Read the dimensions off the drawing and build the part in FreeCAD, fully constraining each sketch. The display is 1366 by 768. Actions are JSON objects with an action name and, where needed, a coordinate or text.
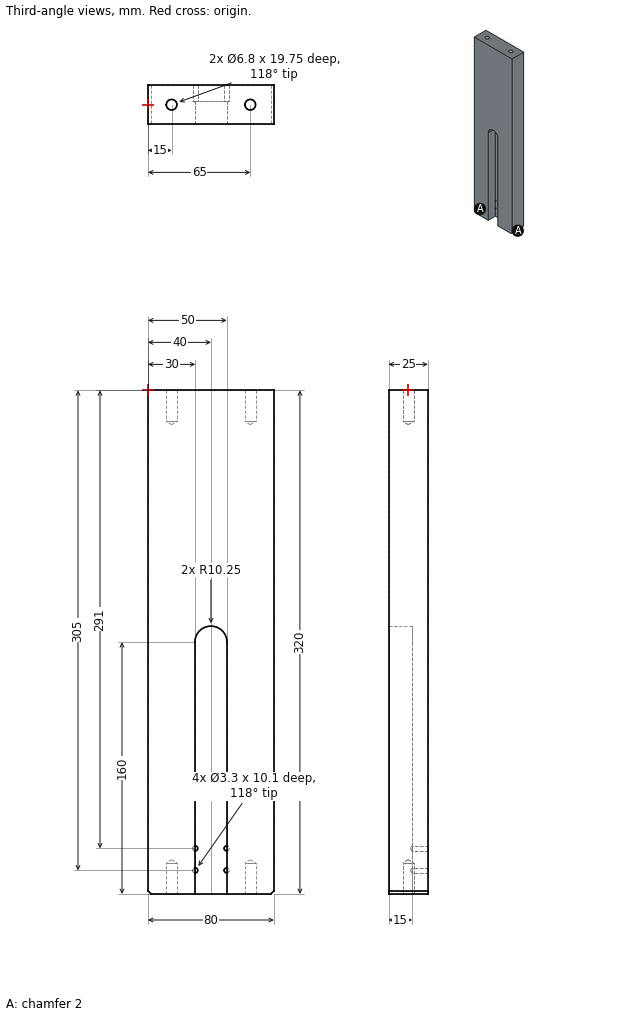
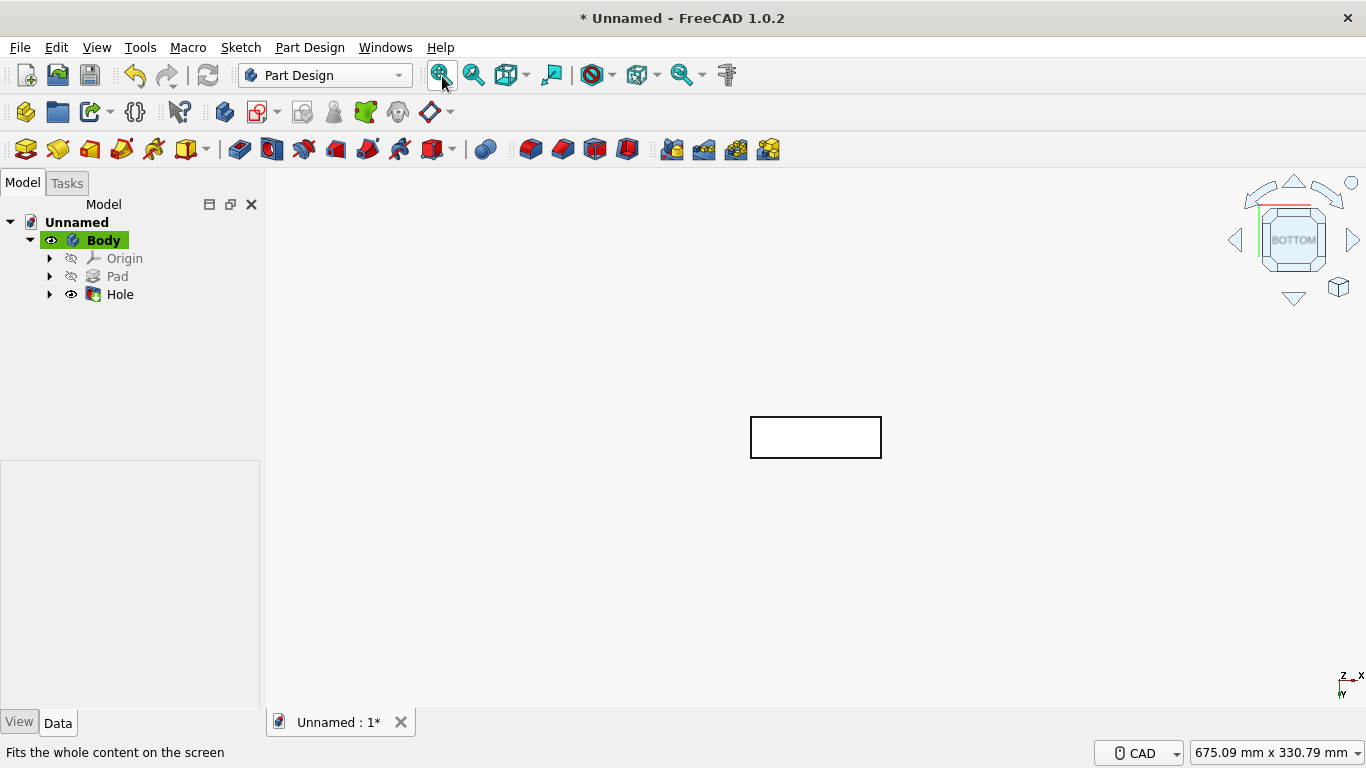
{"action": "key", "text": "v f"}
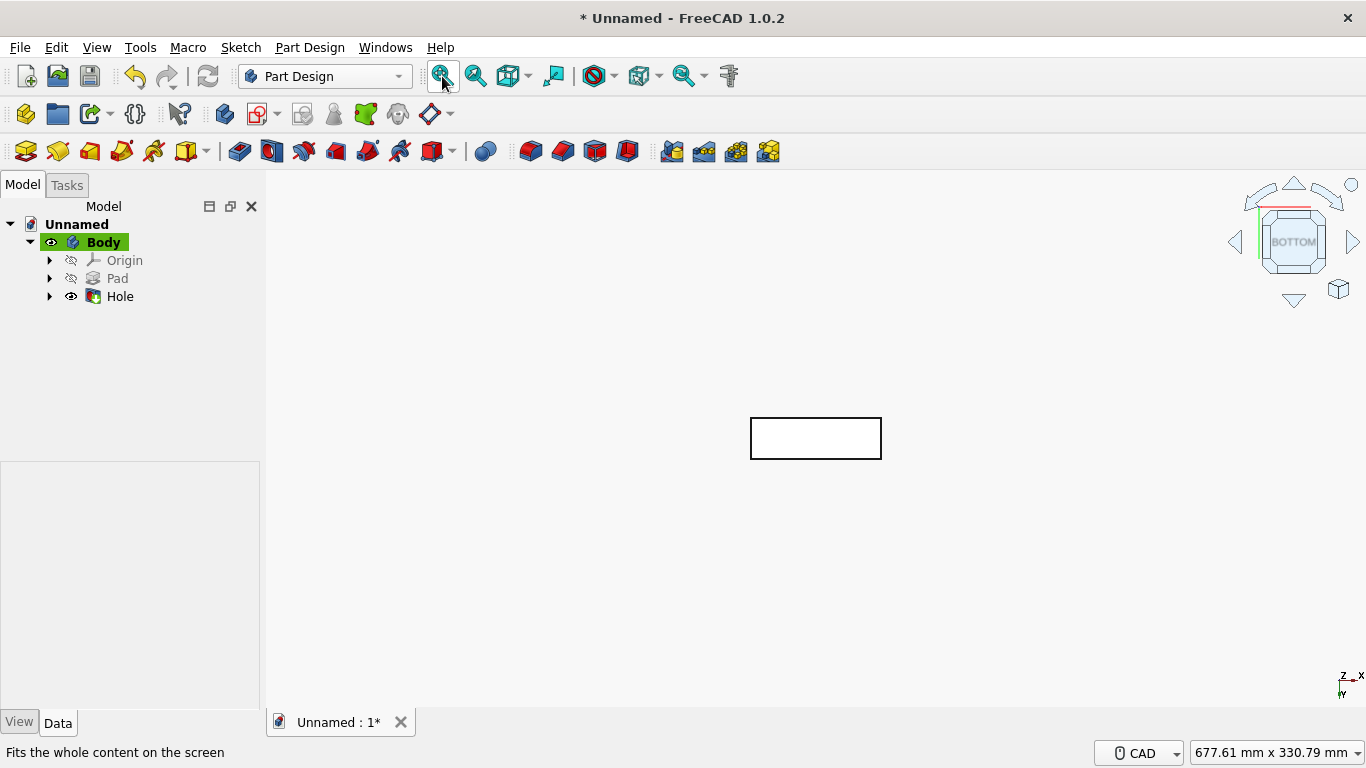
{"action": "left_click", "coordinate": [751, 437]}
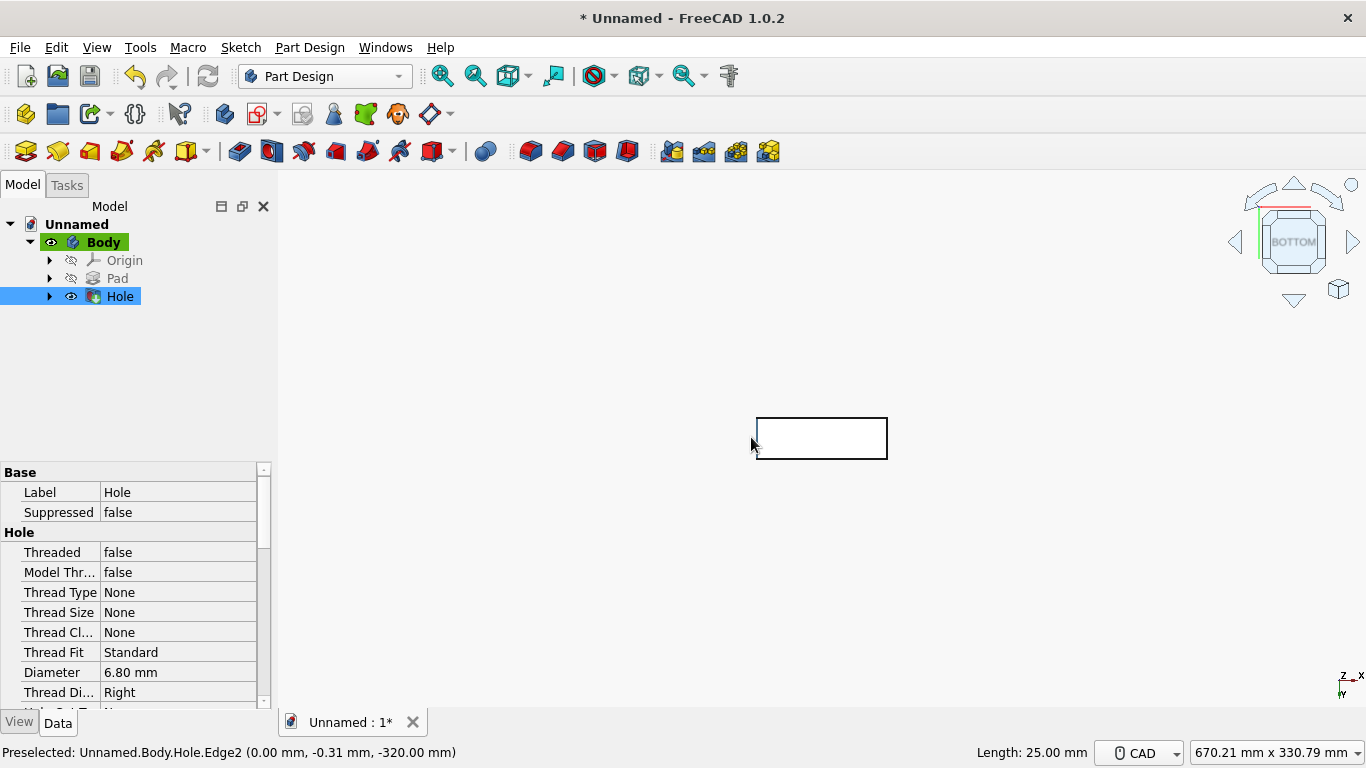
{"action": "left_click", "coordinate": [887, 437], "text": "ctrl"}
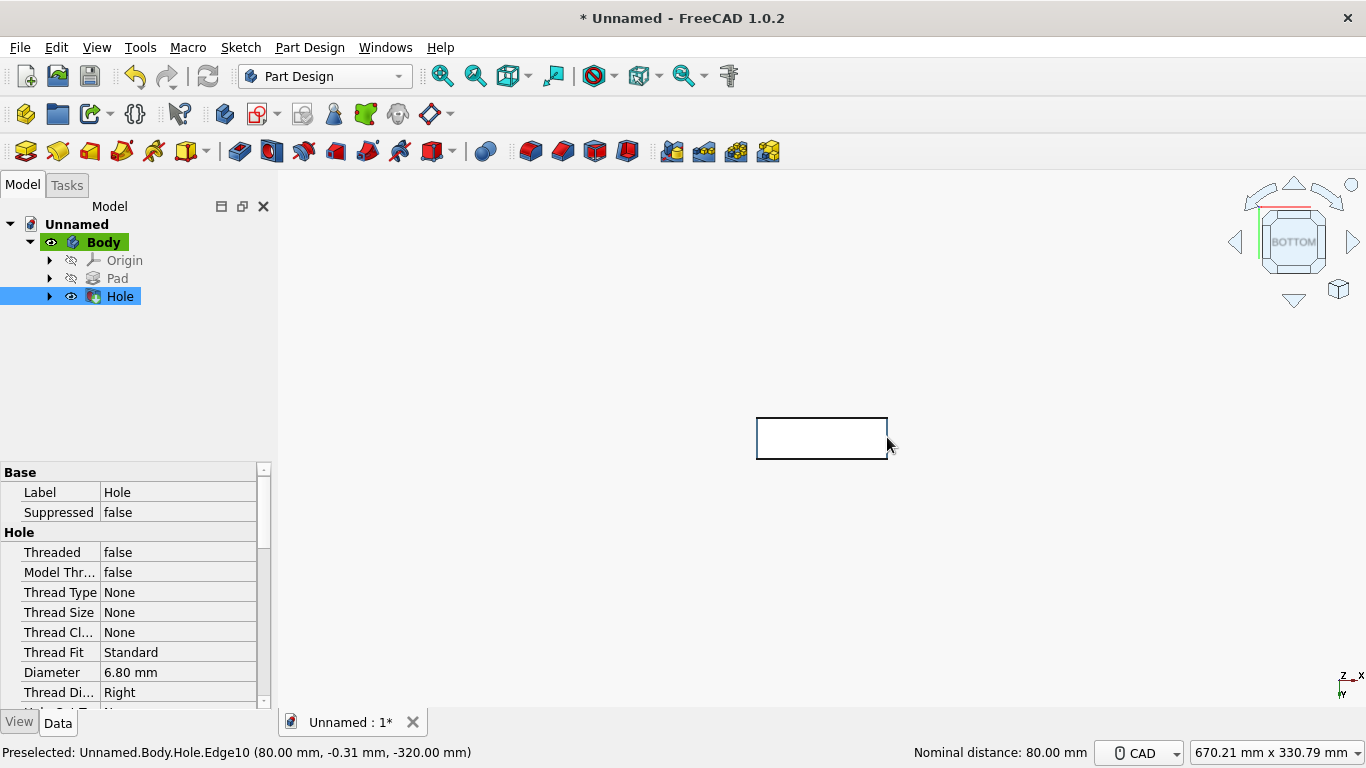
{"action": "left_click", "coordinate": [564, 152]}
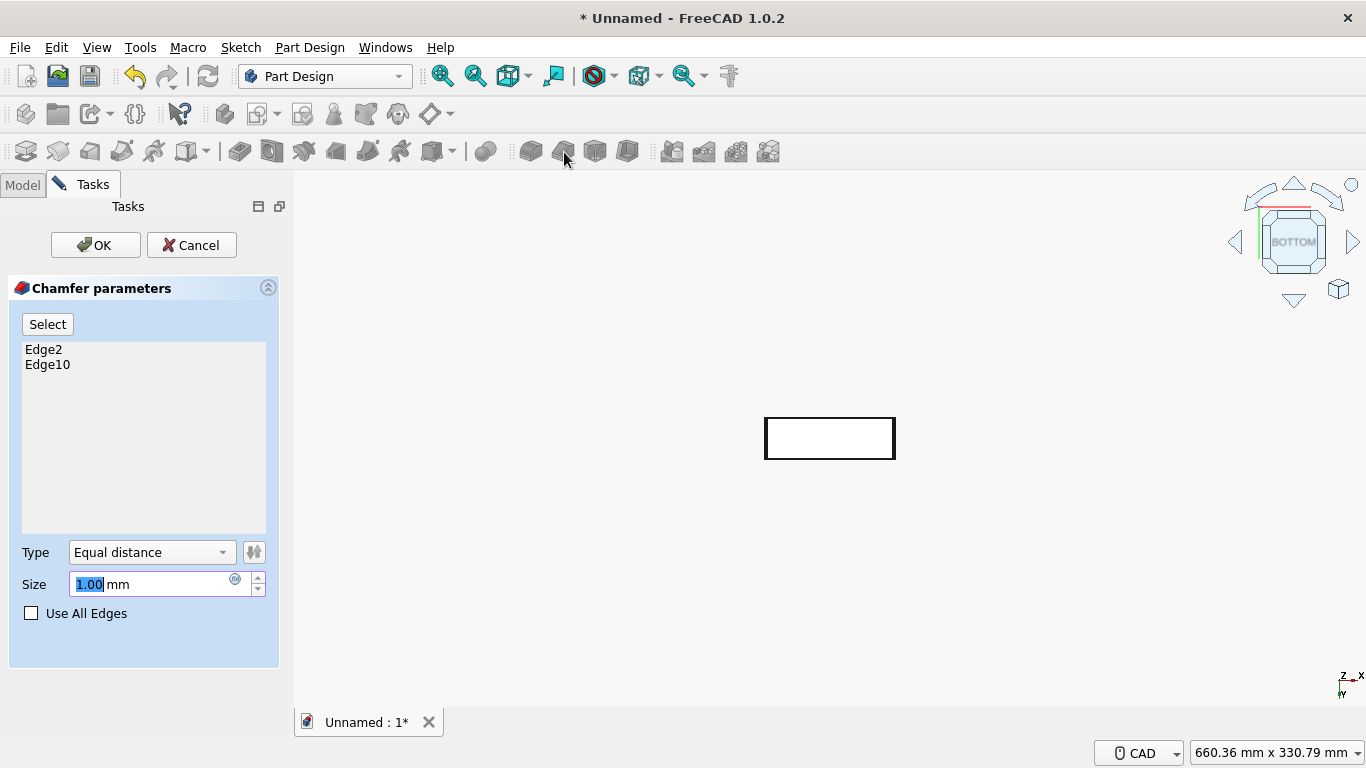
{"action": "type", "text": "2"}
{"action": "key", "text": "Tab"}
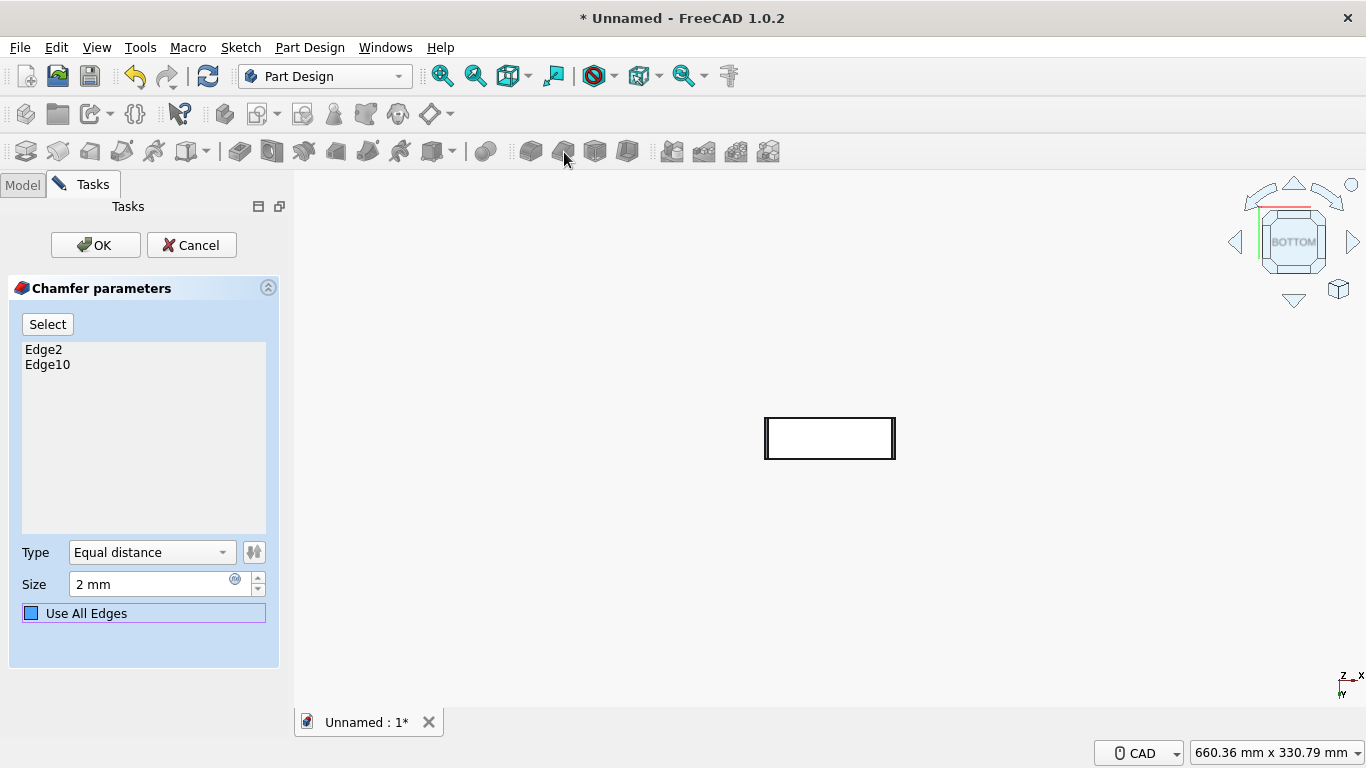
{"action": "left_click", "coordinate": [96, 245]}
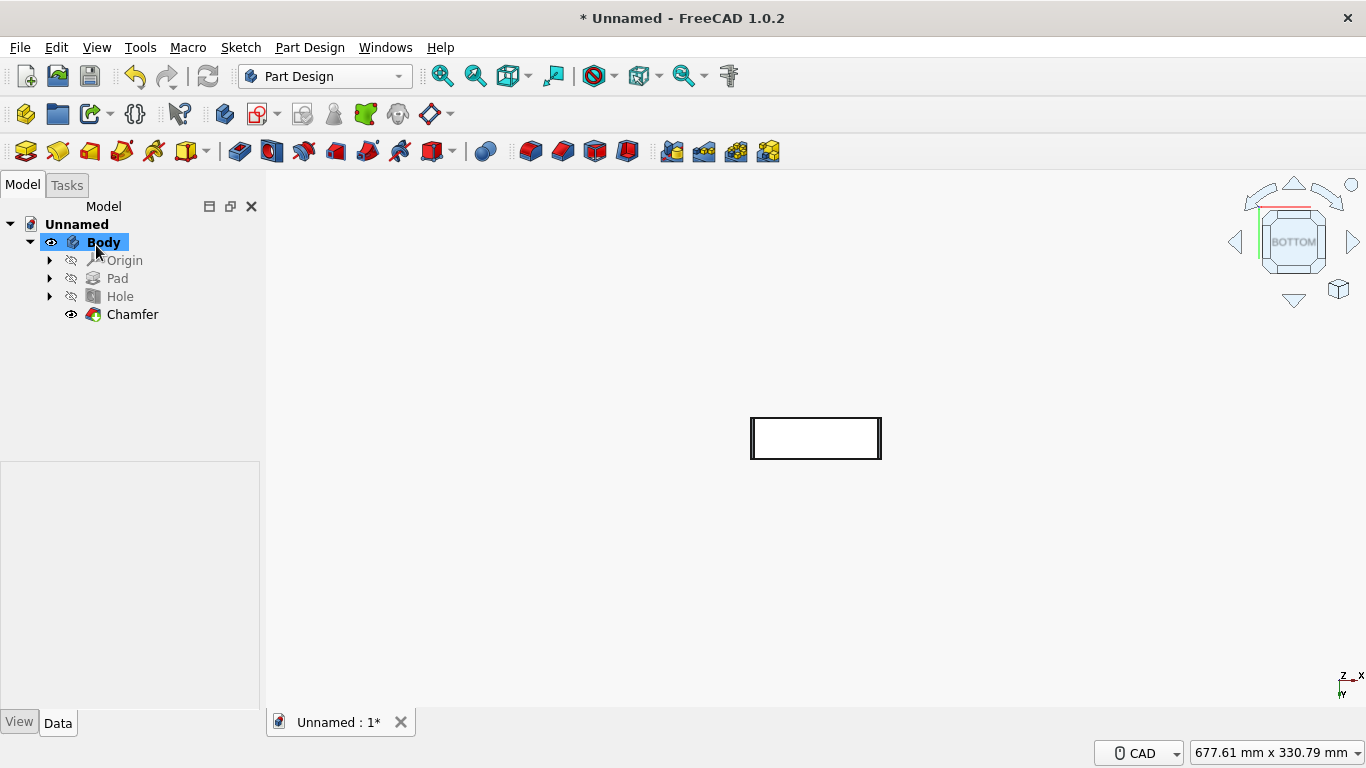
{"action": "key", "text": "v f"}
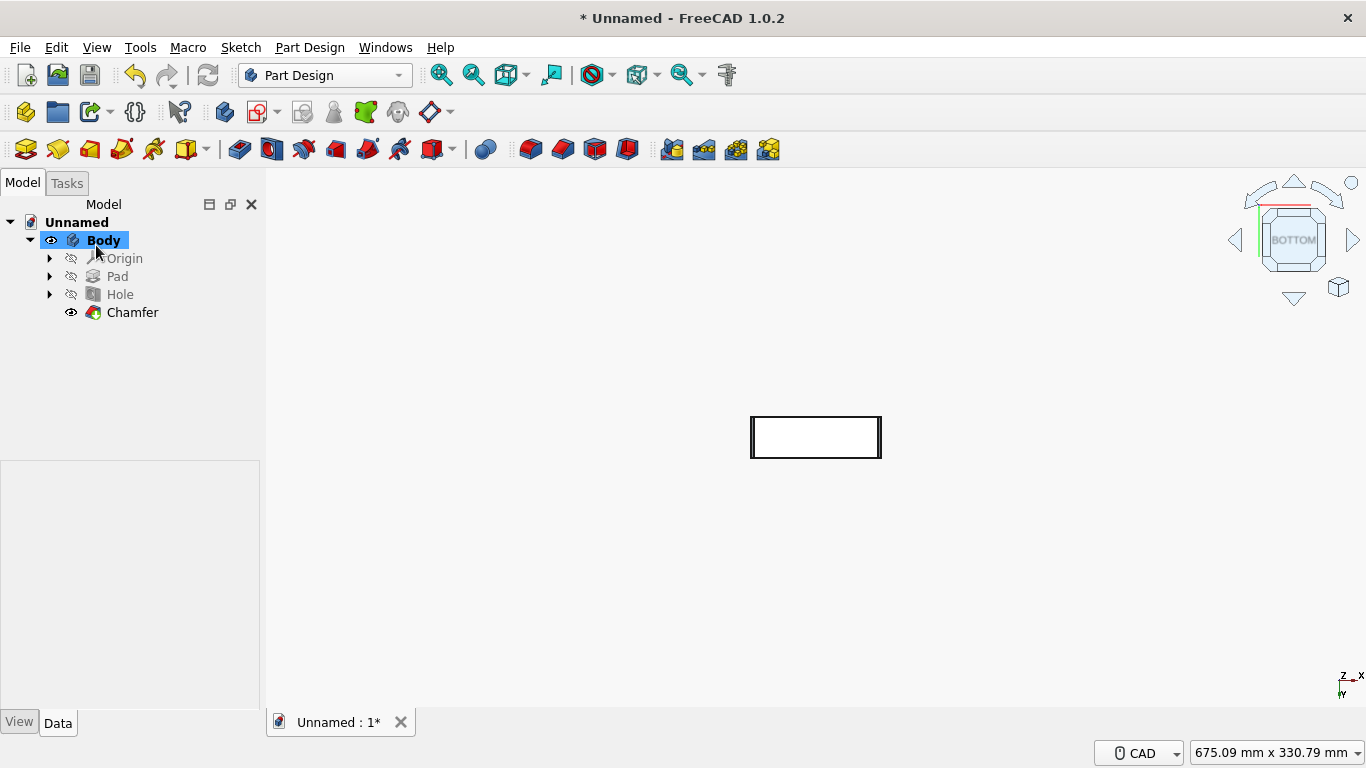
{"action": "key", "text": "4"}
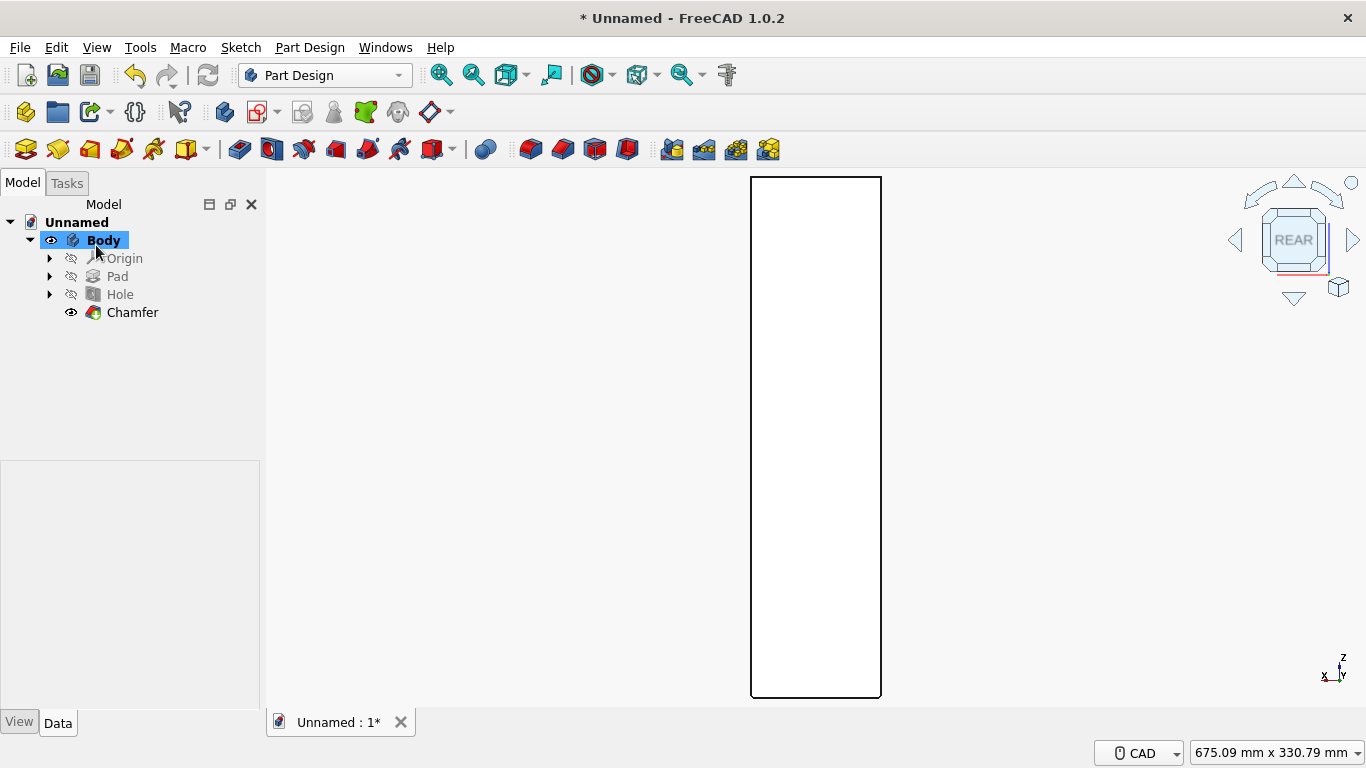
{"action": "left_click", "coordinate": [816, 288]}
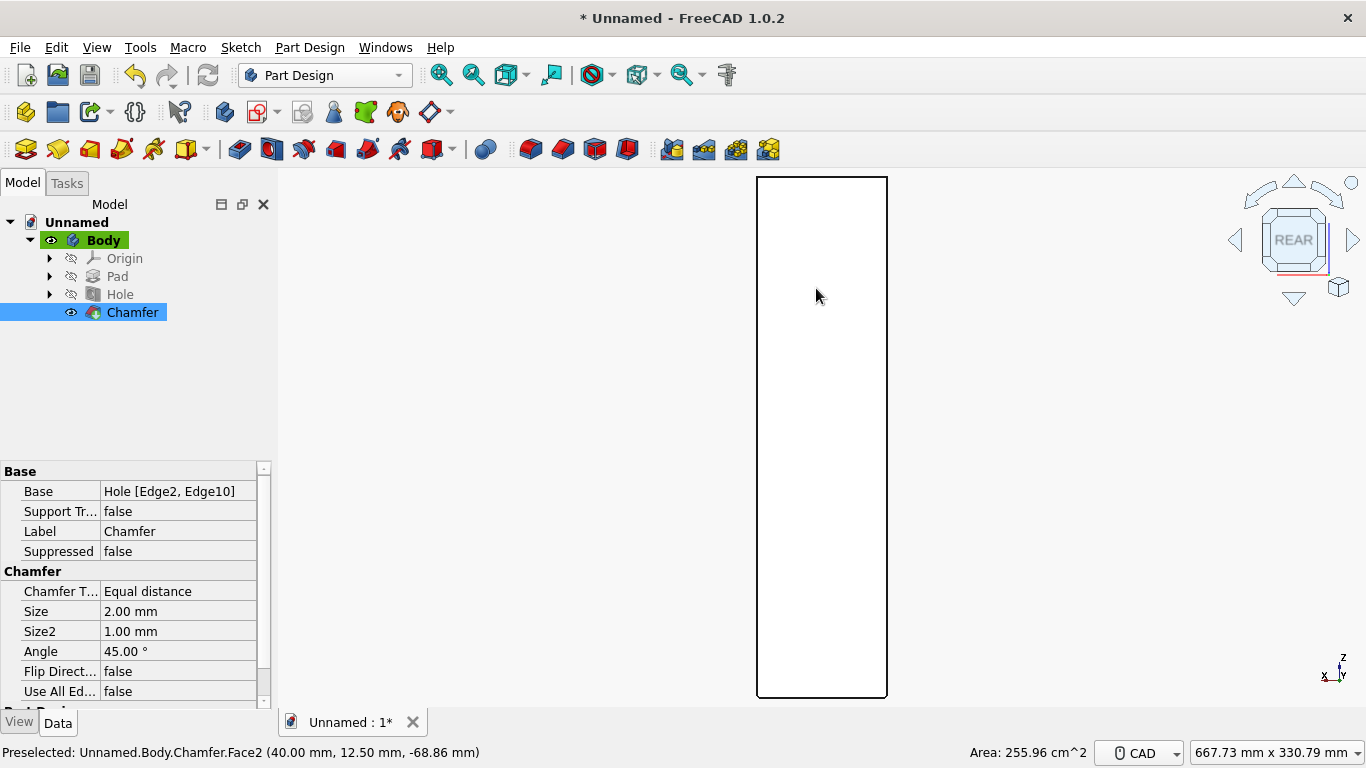
{"action": "left_click", "coordinate": [258, 112]}